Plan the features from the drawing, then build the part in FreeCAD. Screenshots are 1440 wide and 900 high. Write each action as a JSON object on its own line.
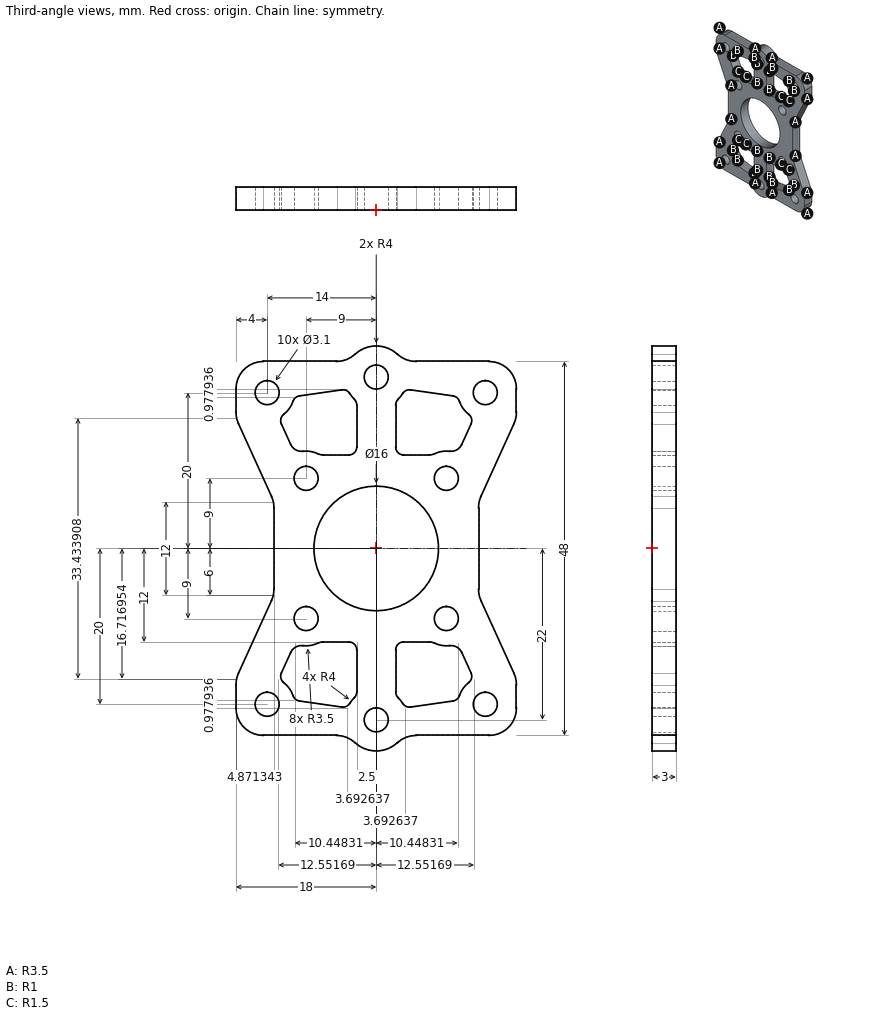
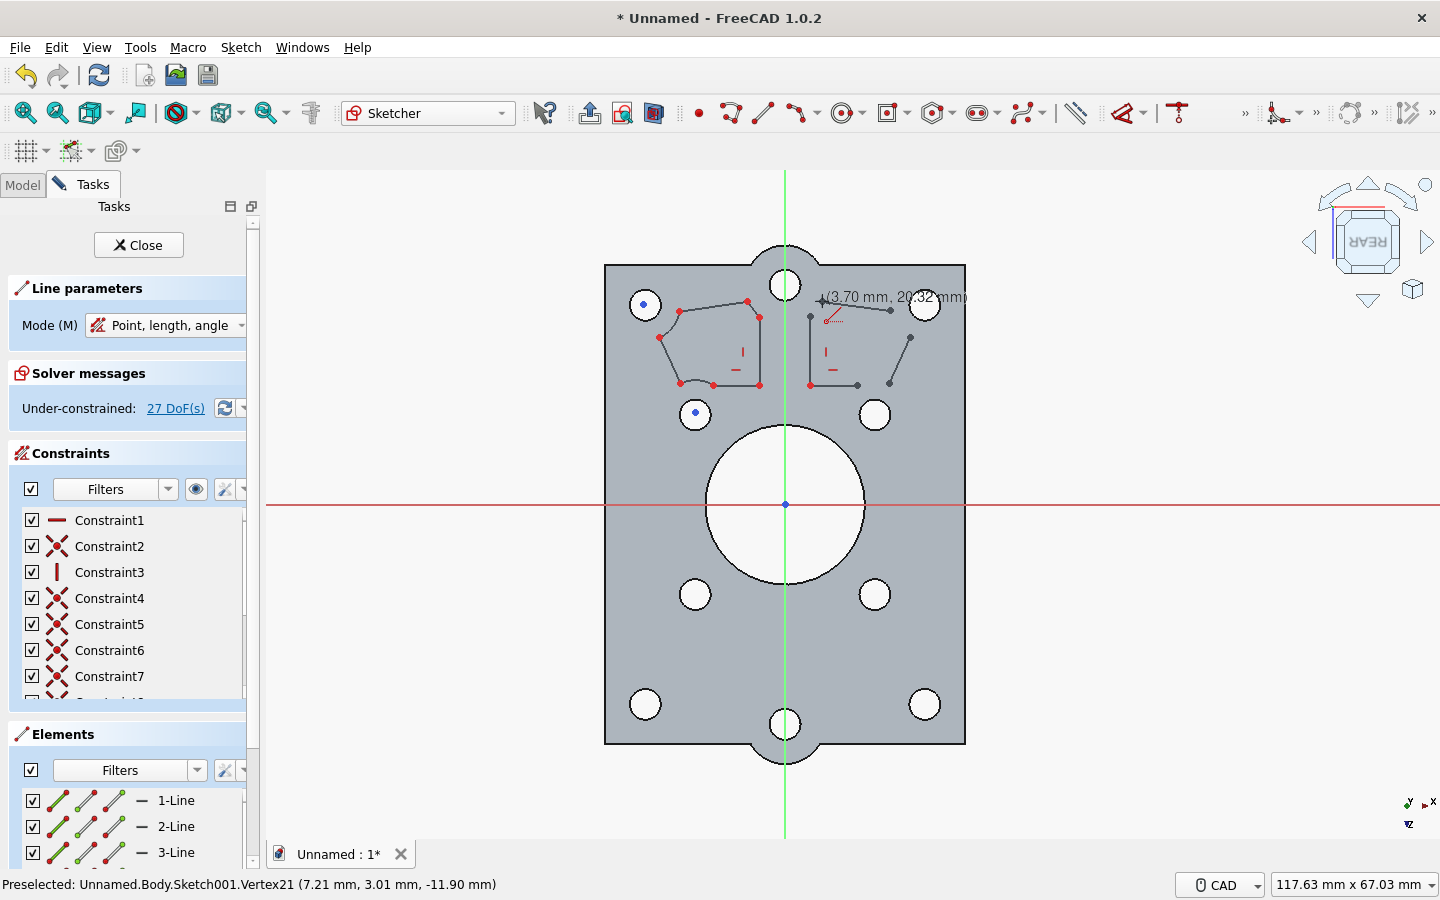
{"action": "left_click", "coordinate": [796, 114]}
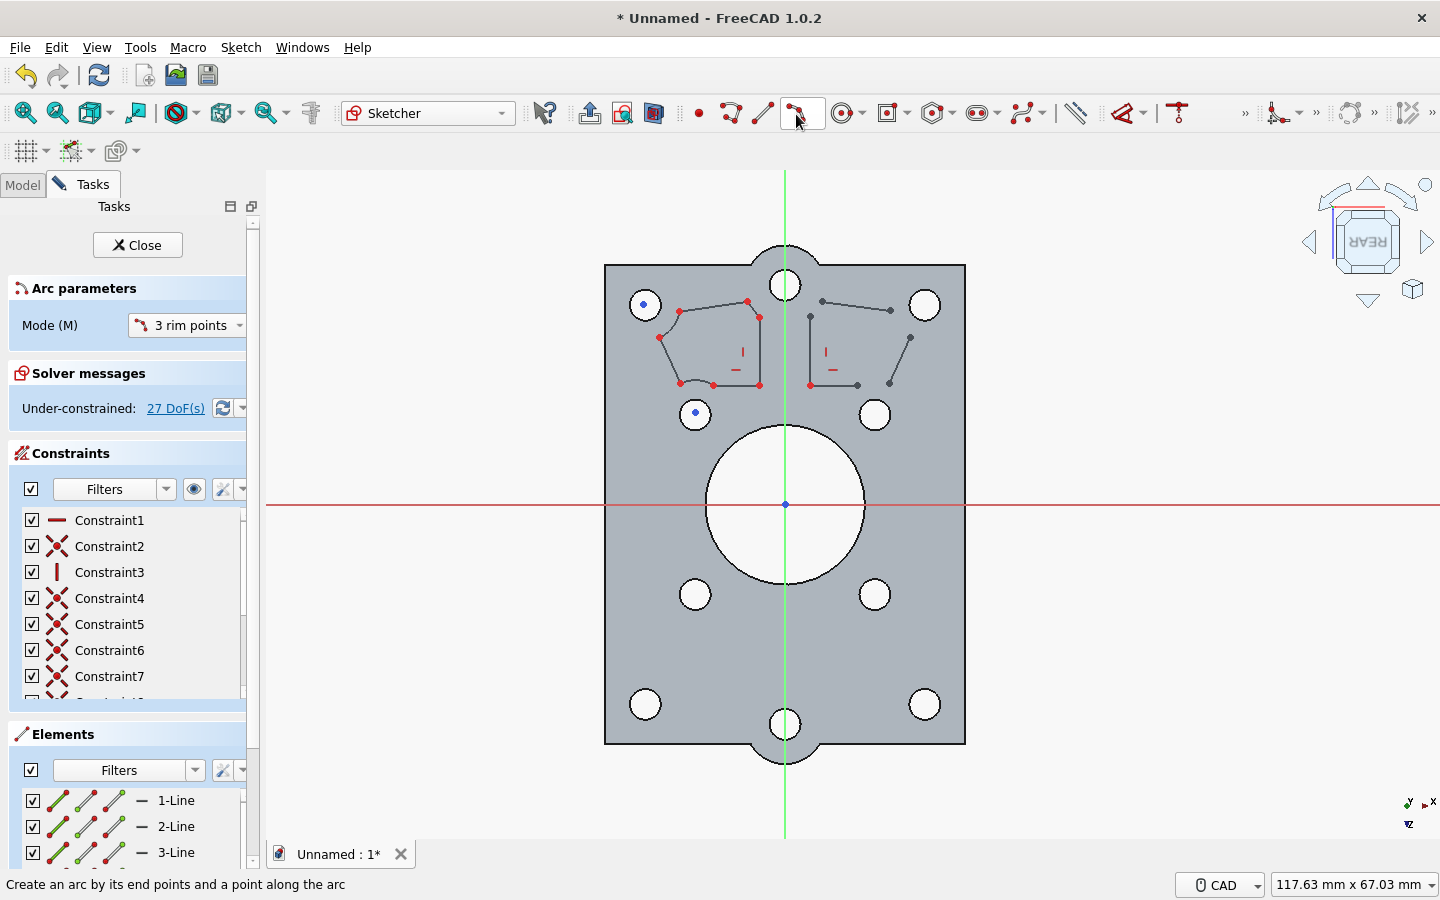
{"action": "left_click", "coordinate": [857, 386]}
{"action": "left_click", "coordinate": [889, 384]}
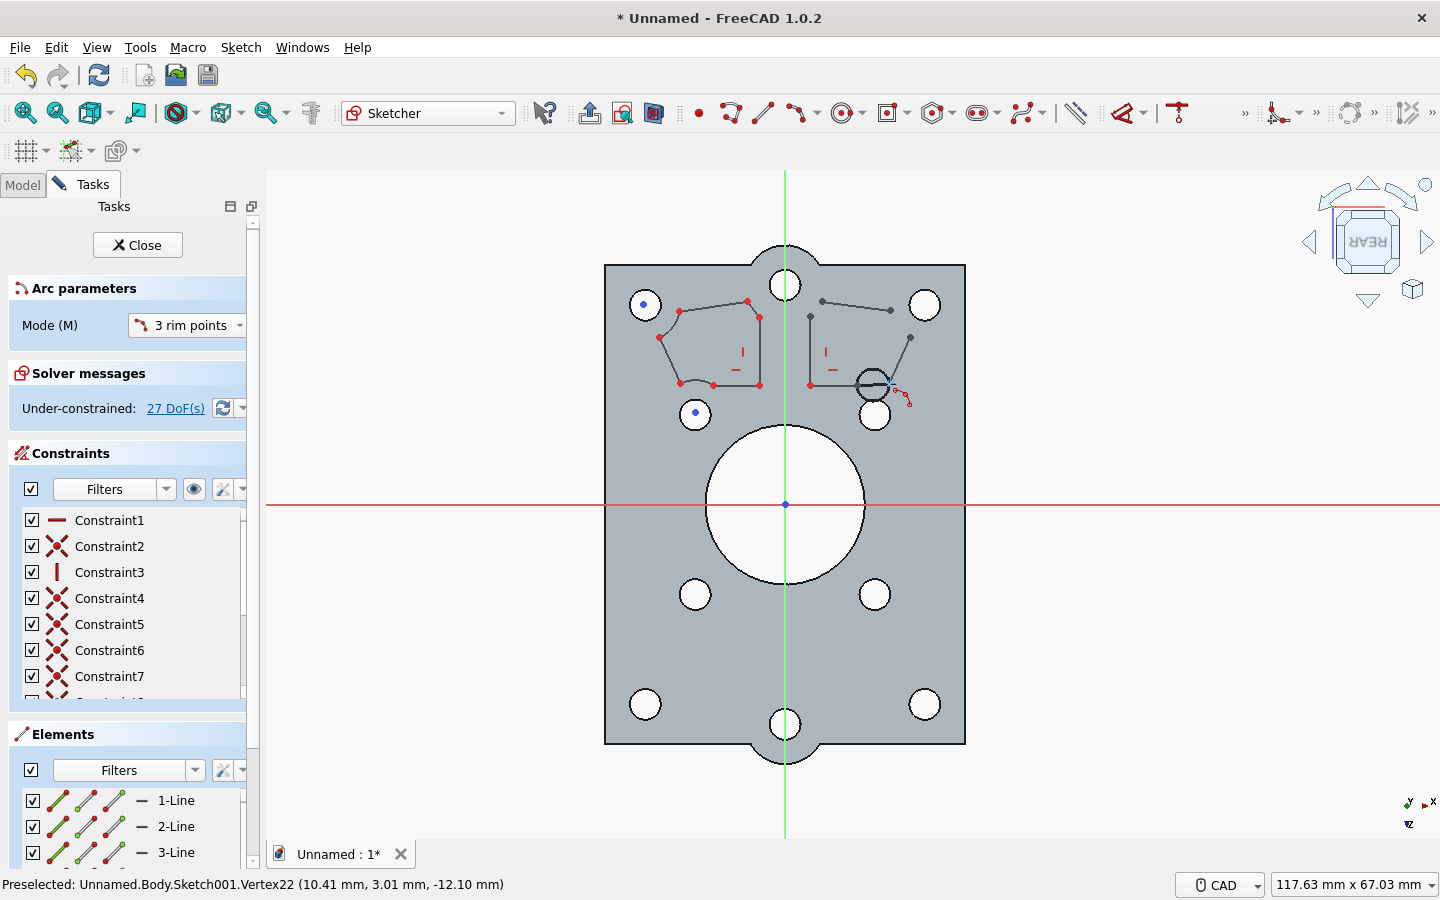
{"action": "scroll", "coordinate": [873, 380], "scroll_direction": "up", "scroll_amount": 7}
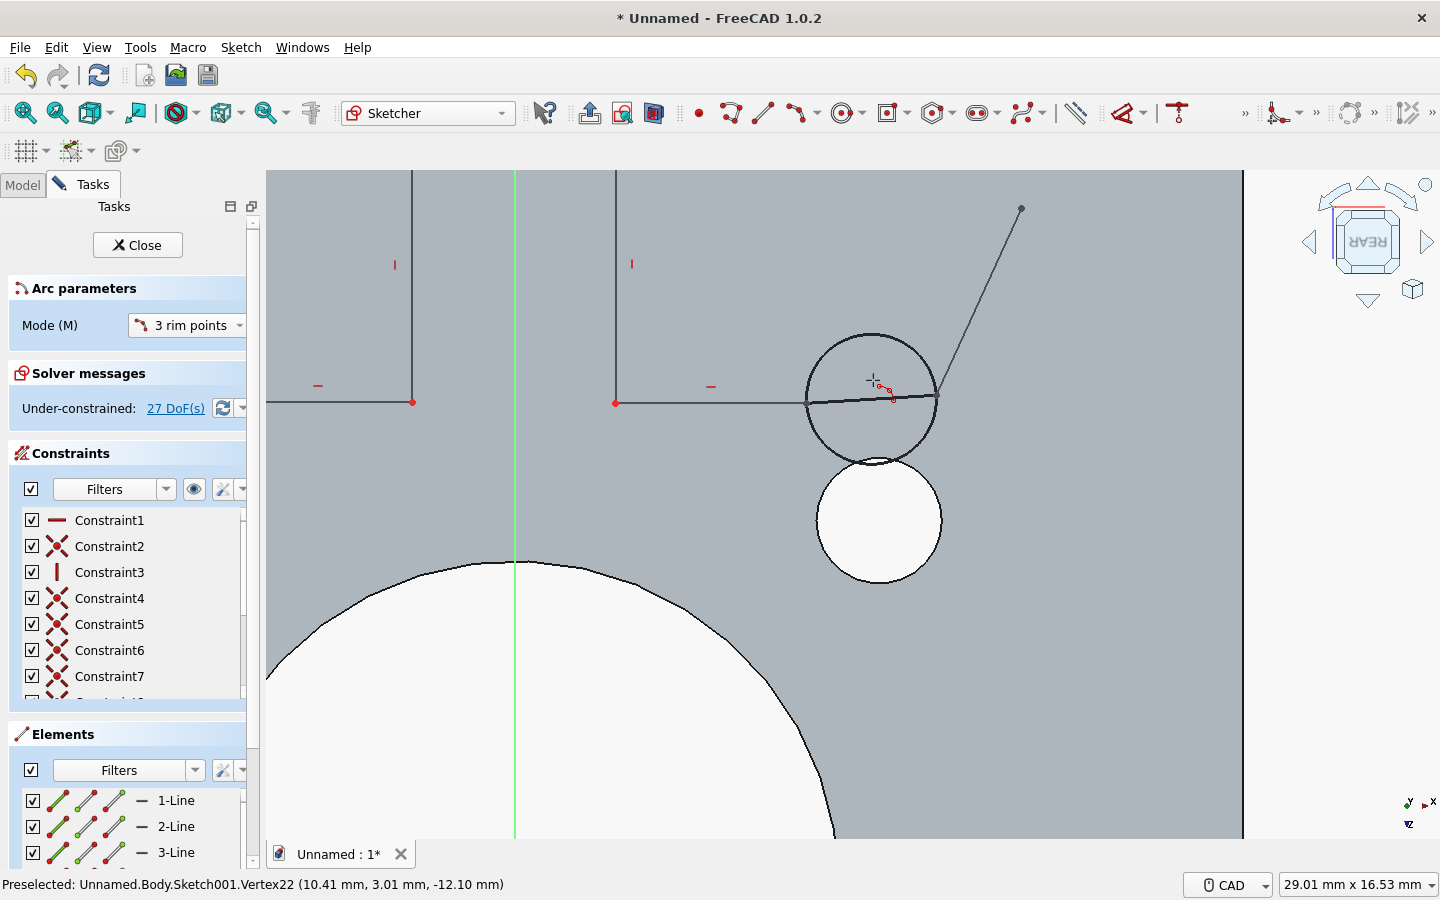
{"action": "left_click", "coordinate": [871, 379]}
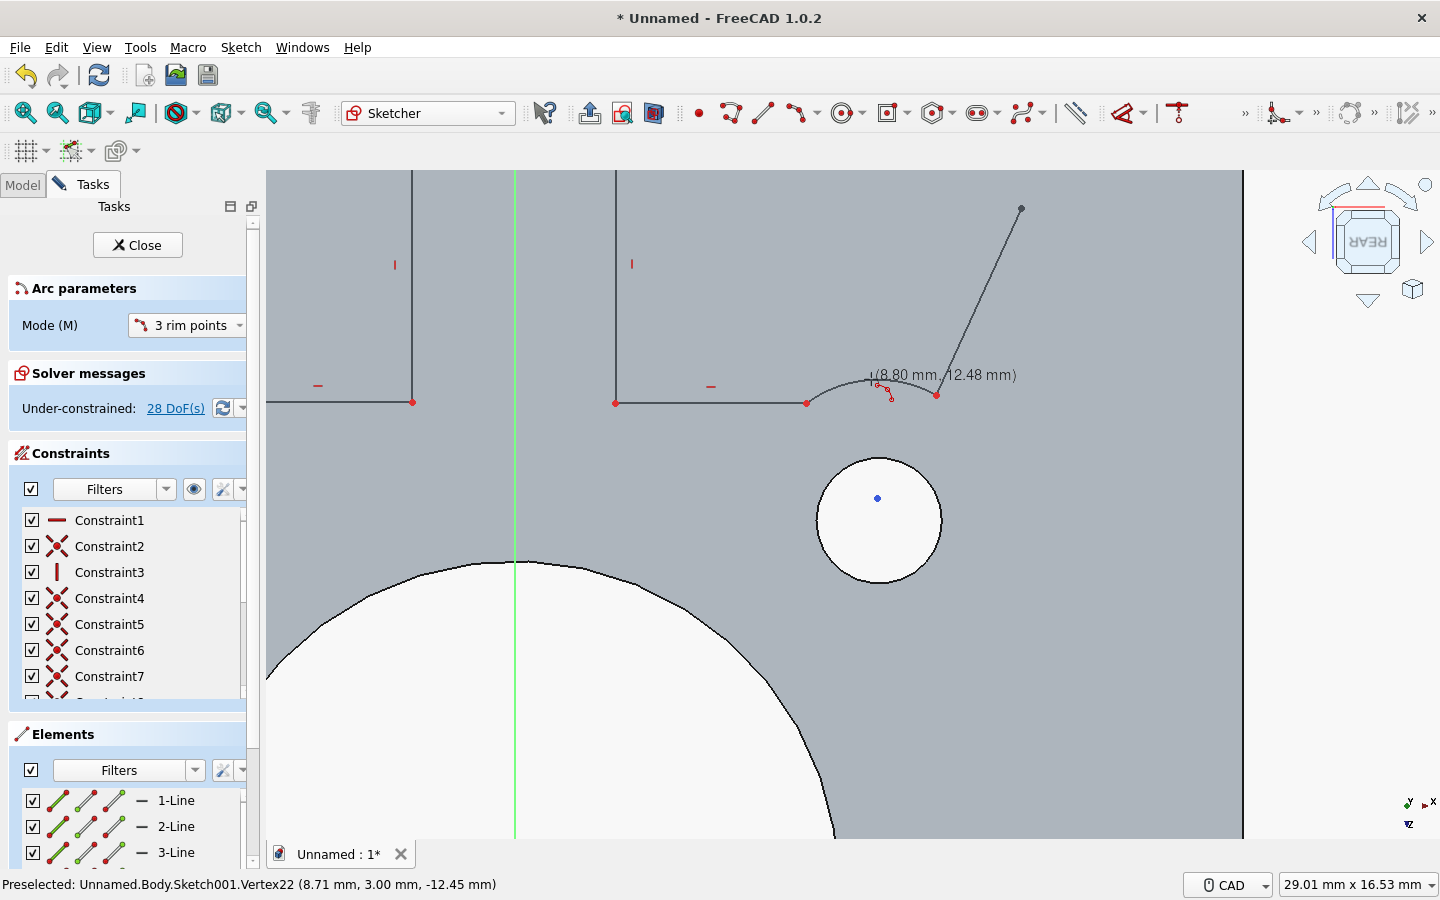
{"action": "scroll", "coordinate": [873, 380], "scroll_direction": "down", "scroll_amount": 7}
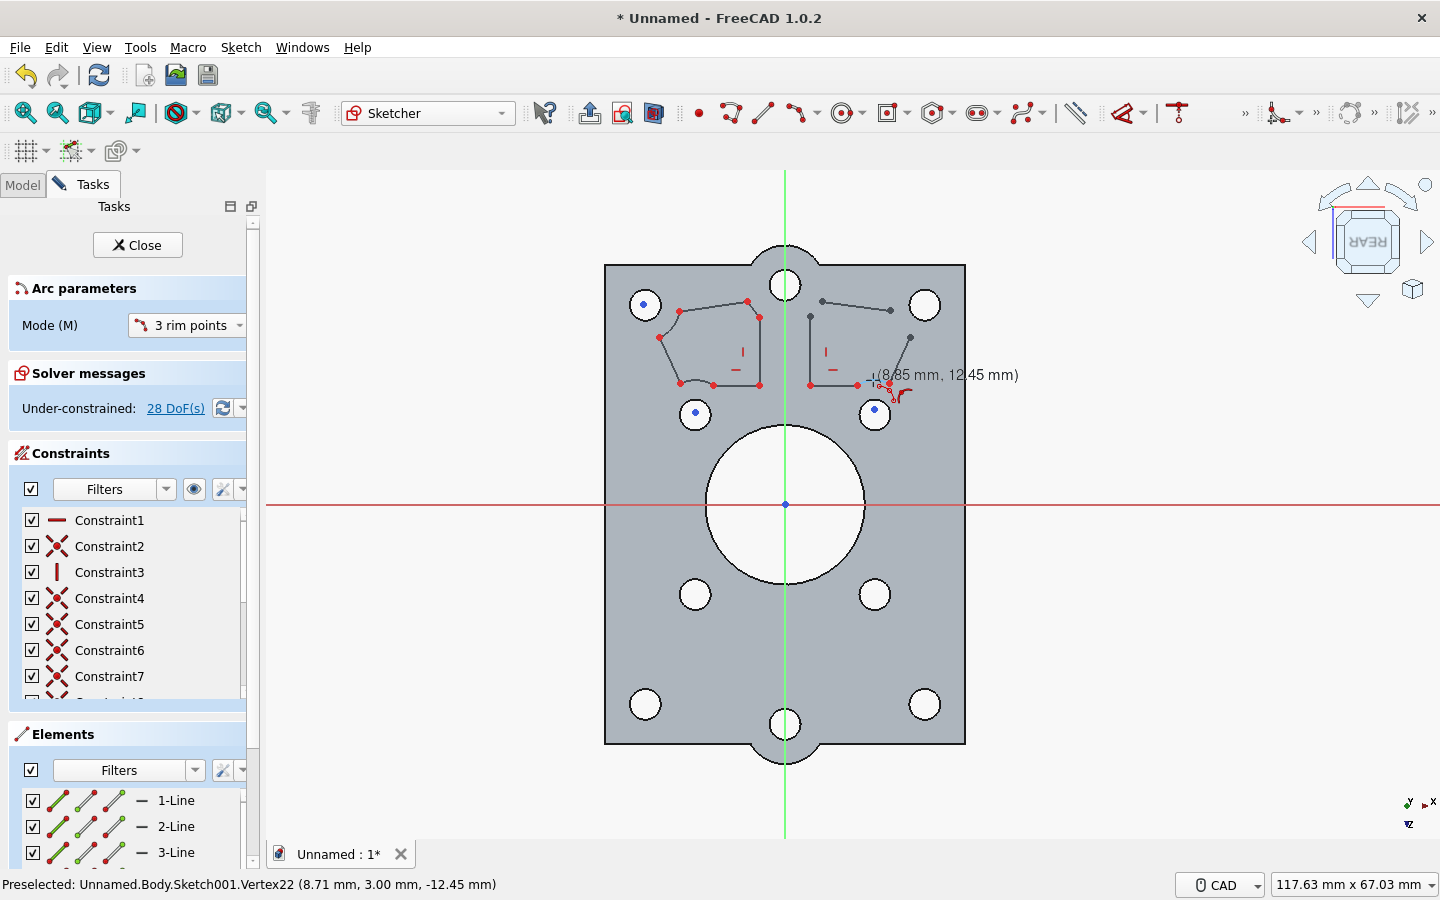
{"action": "left_click", "coordinate": [910, 338]}
{"action": "left_click", "coordinate": [890, 311]}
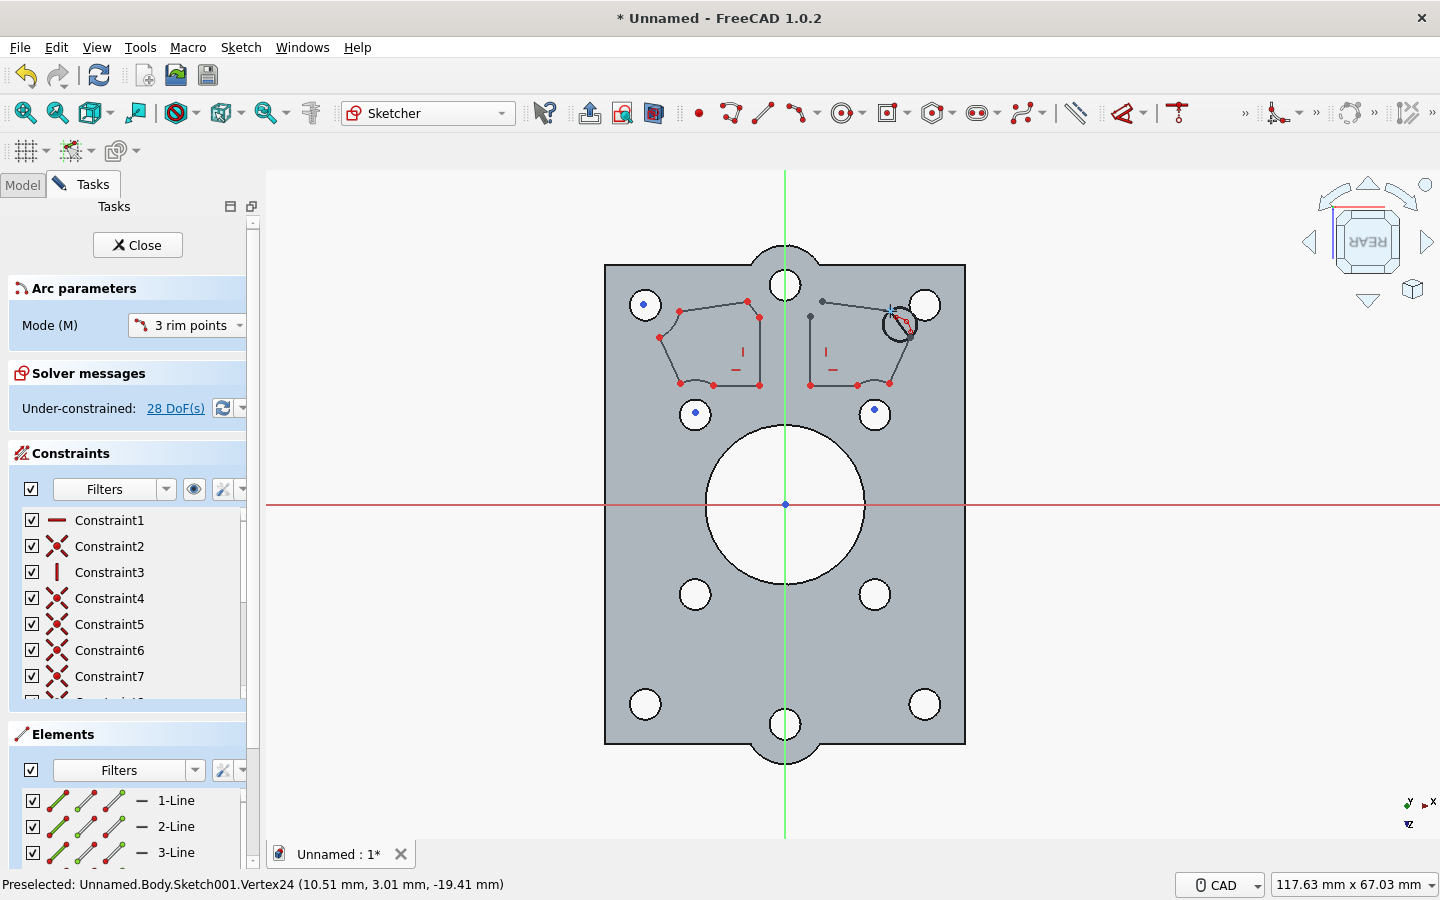
{"action": "scroll", "coordinate": [897, 326], "scroll_direction": "up", "scroll_amount": 7}